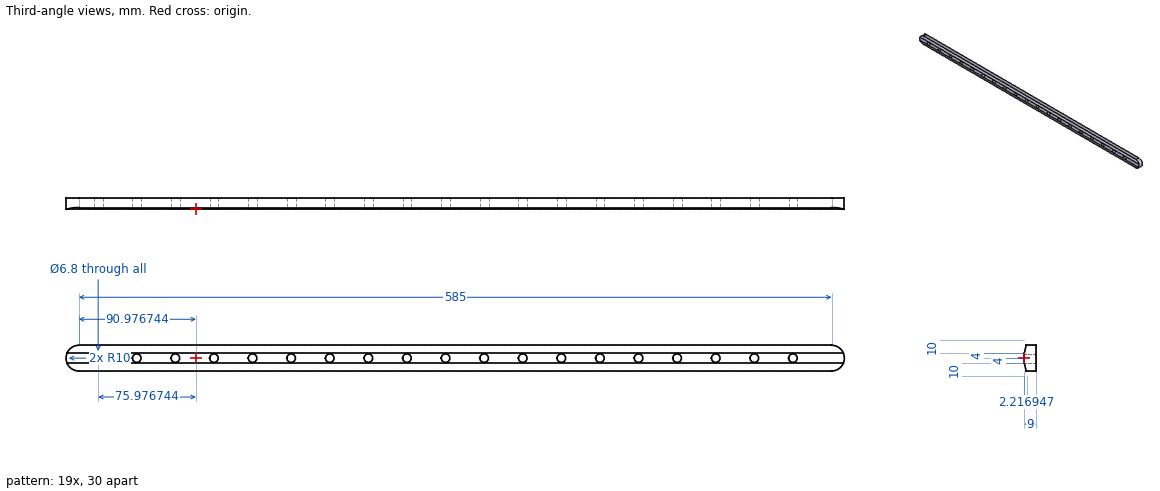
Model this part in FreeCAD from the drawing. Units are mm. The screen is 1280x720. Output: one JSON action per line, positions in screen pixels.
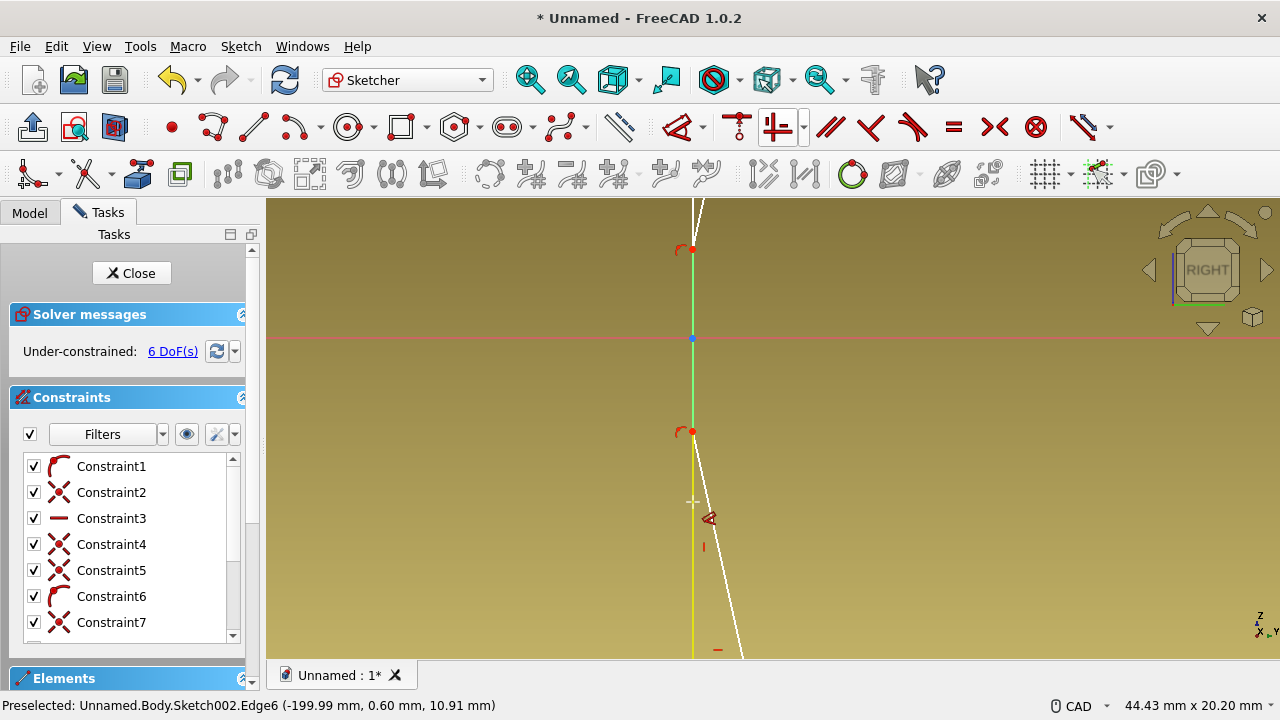
{"action": "left_click", "coordinate": [693, 500]}
{"action": "left_click", "coordinate": [659, 531]}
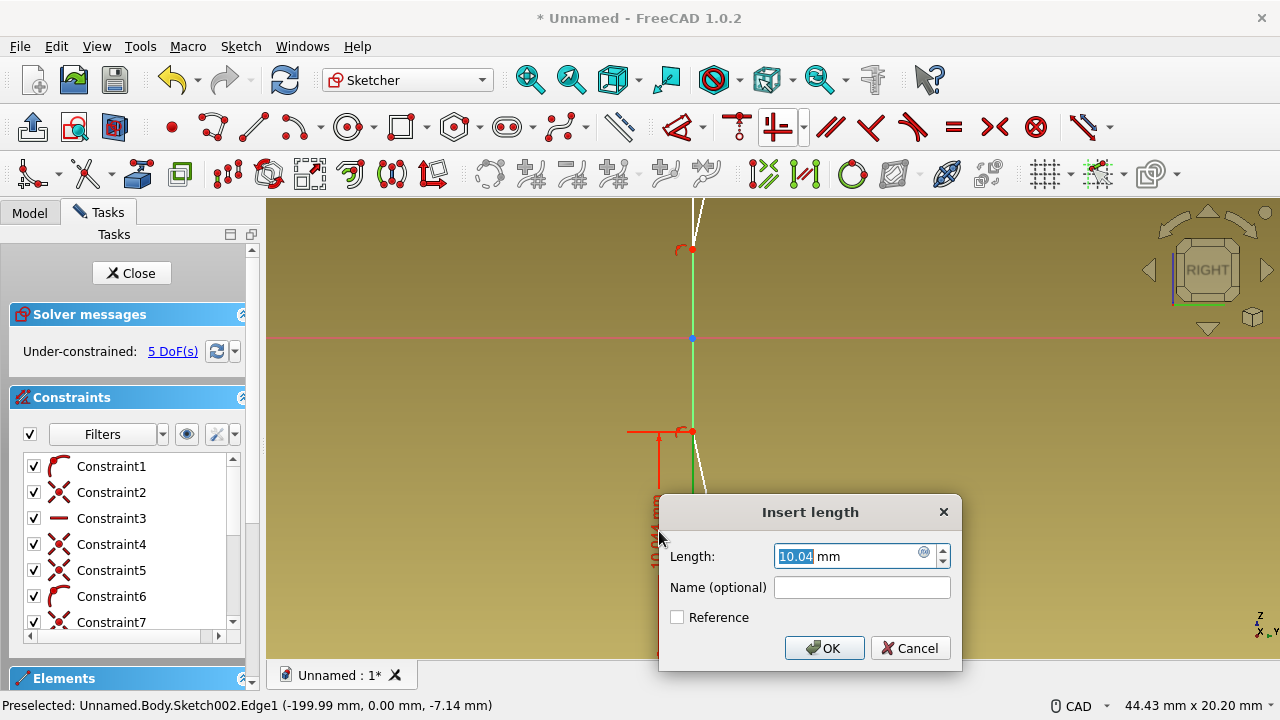
{"action": "type", "text": "10"}
{"action": "key", "text": "Return"}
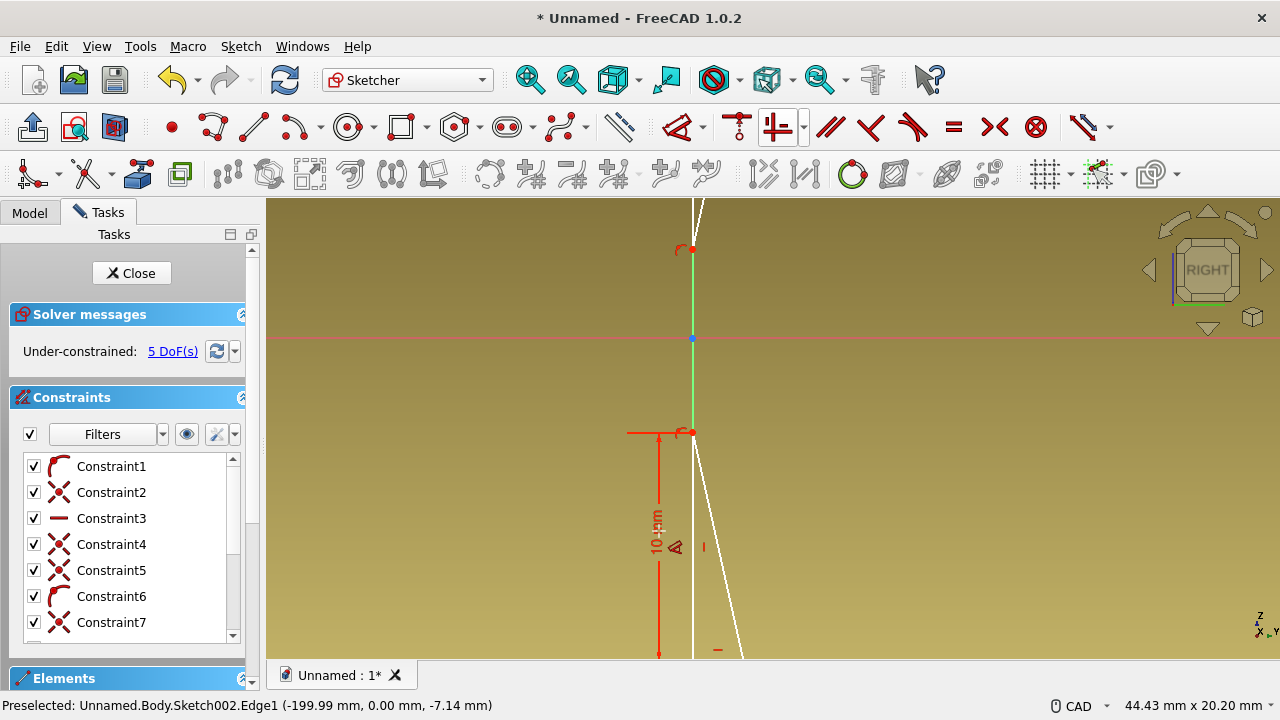
{"action": "scroll", "coordinate": [693, 502], "scroll_direction": "down", "scroll_amount": 4}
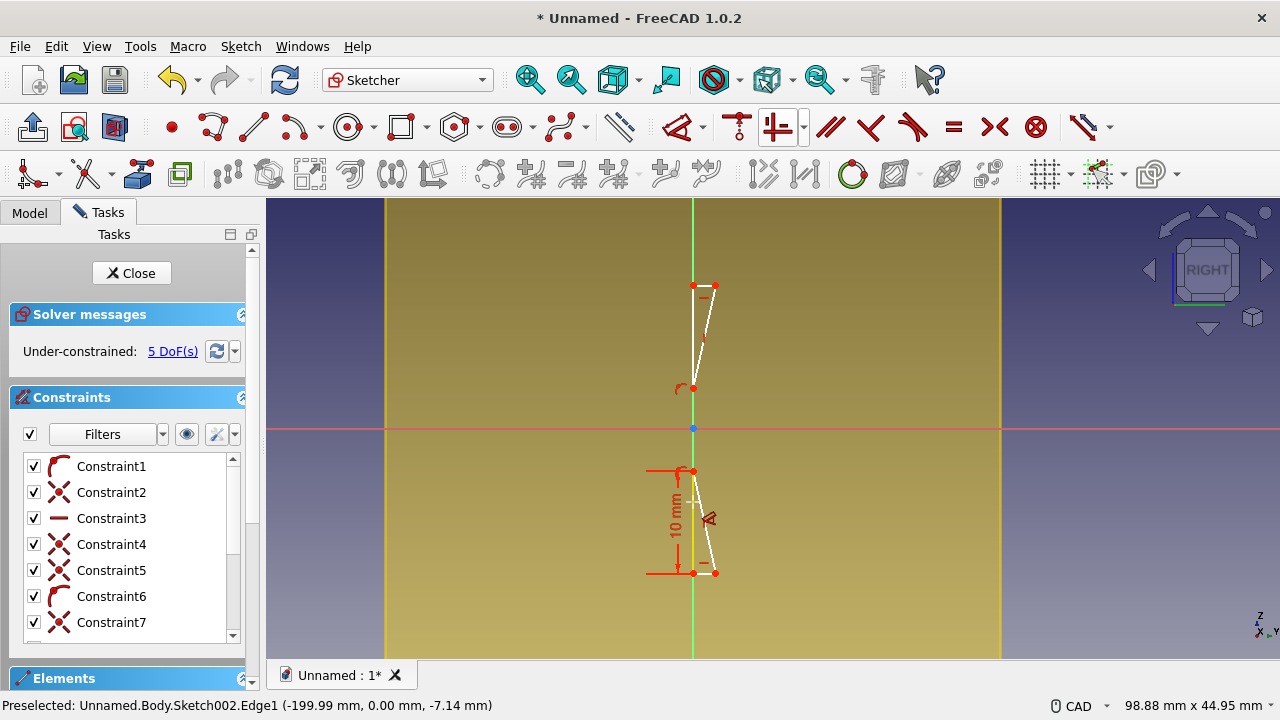
{"action": "left_click", "coordinate": [693, 317]}
{"action": "left_click", "coordinate": [659, 337]}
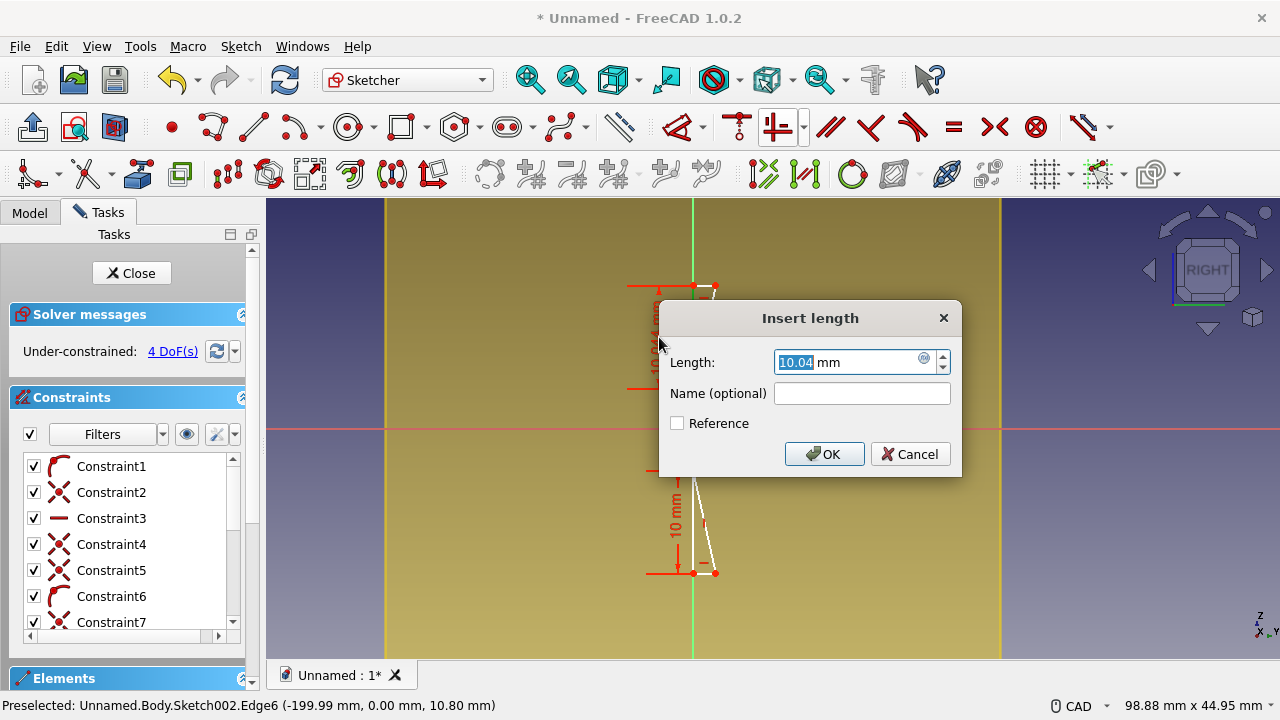
{"action": "type", "text": "10"}
{"action": "key", "text": "Return"}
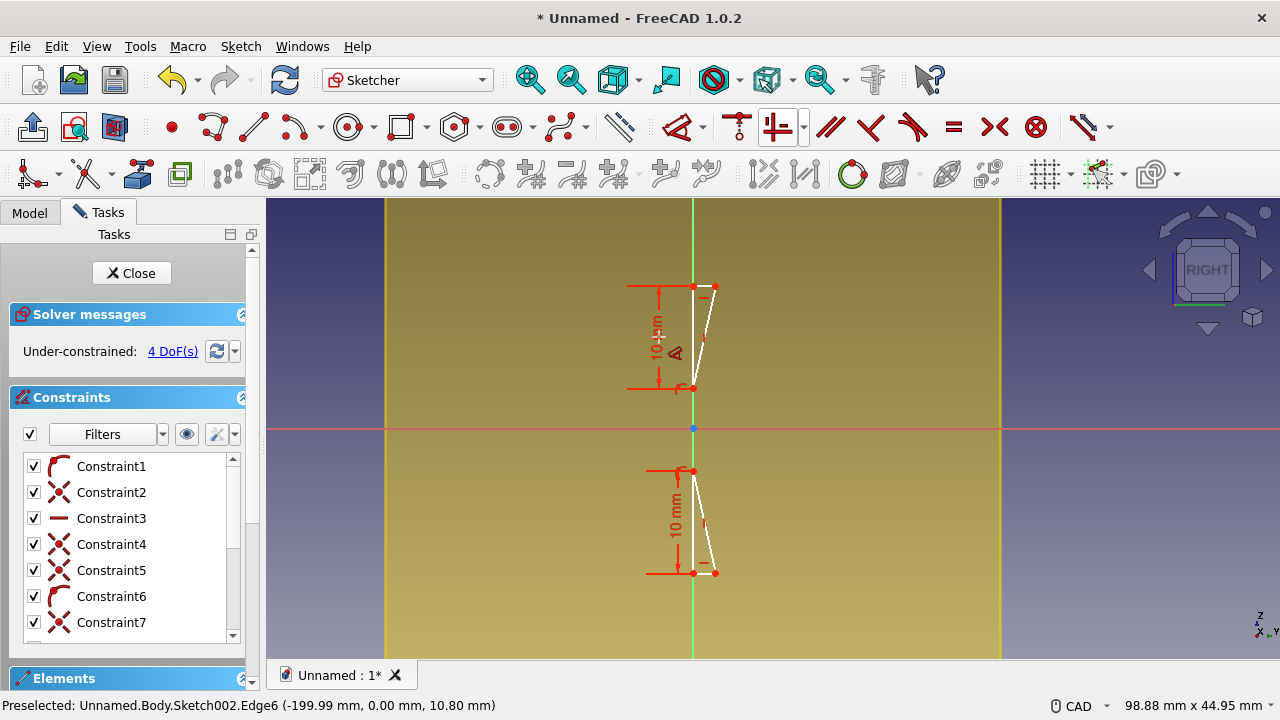
{"action": "left_click", "coordinate": [693, 471]}
{"action": "left_click", "coordinate": [659, 450]}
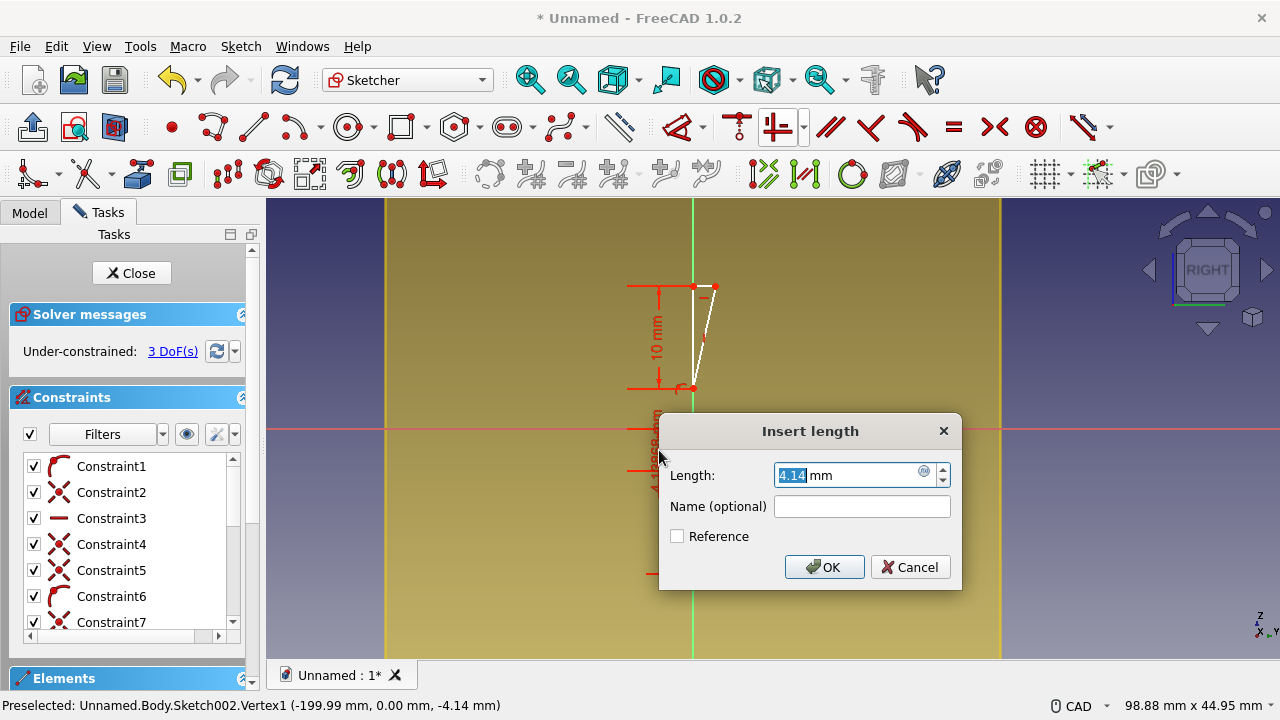
{"action": "type", "text": "4"}
{"action": "key", "text": "Return"}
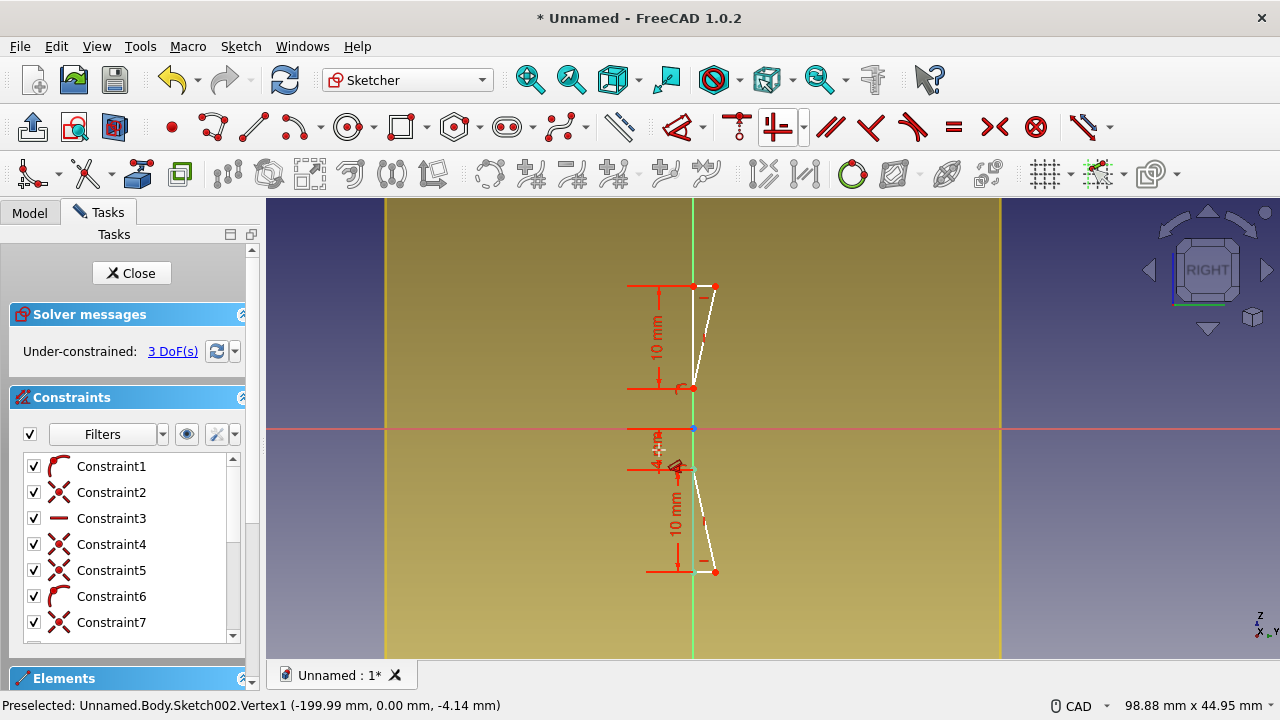
{"action": "left_click", "coordinate": [693, 389]}
{"action": "left_click", "coordinate": [659, 409]}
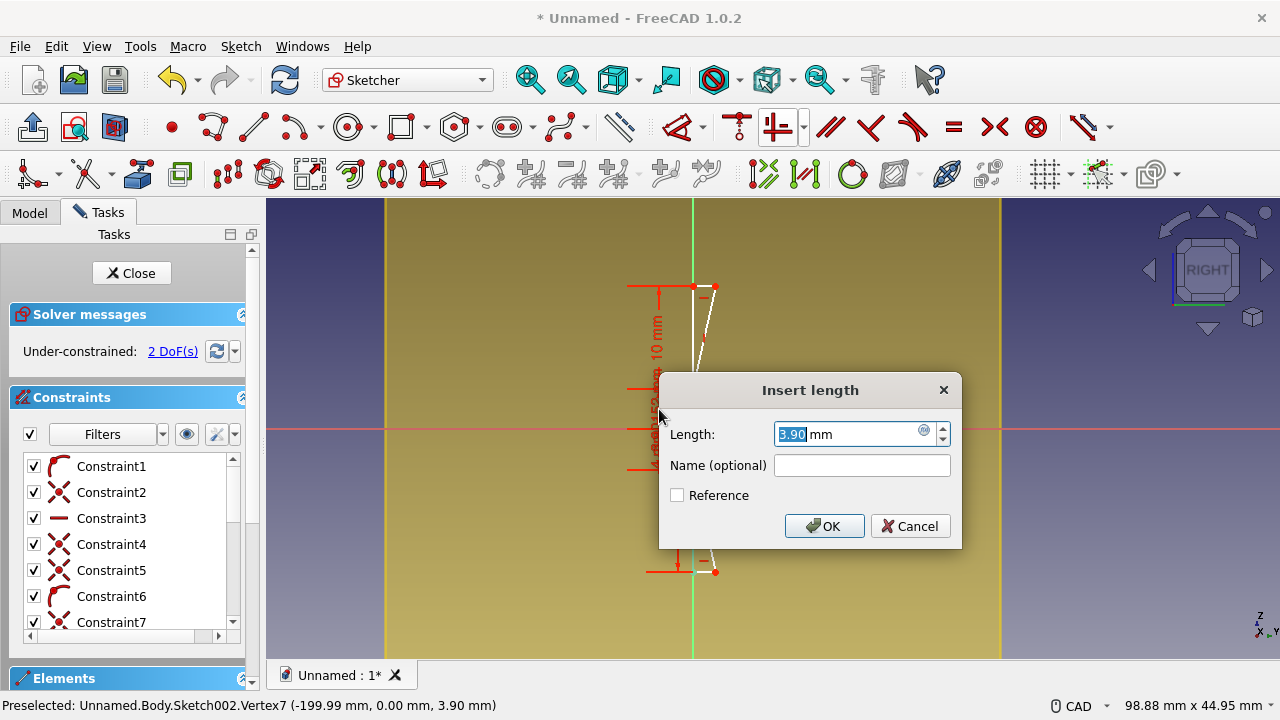
{"action": "type", "text": "4"}
{"action": "key", "text": "Return"}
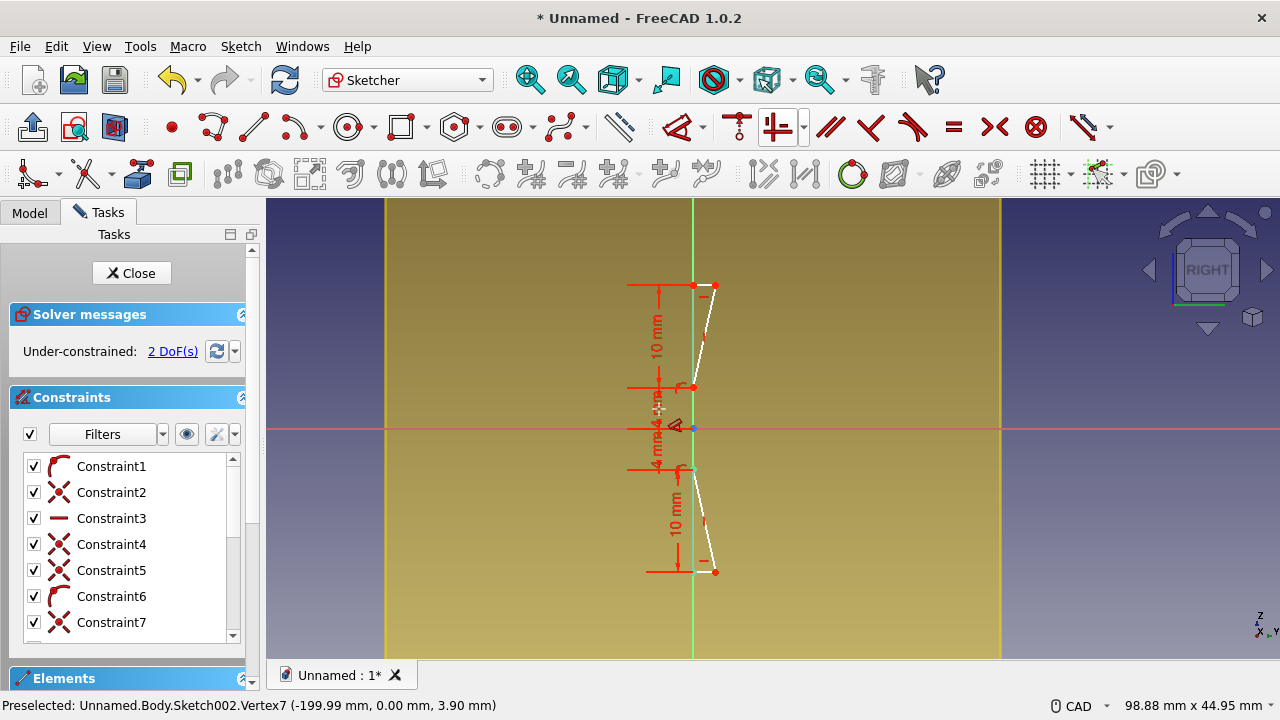
{"action": "scroll", "coordinate": [702, 572], "scroll_direction": "up", "scroll_amount": 3}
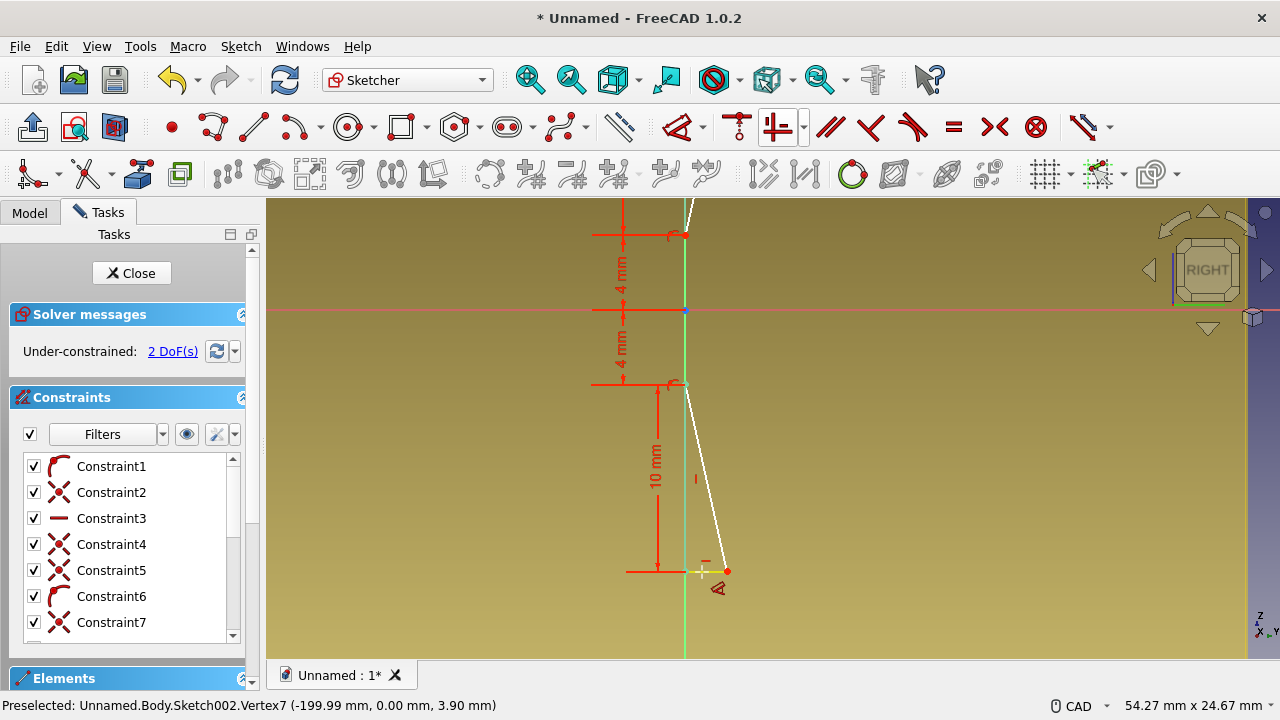
{"action": "left_click", "coordinate": [702, 572]}
{"action": "left_click", "coordinate": [706, 606]}